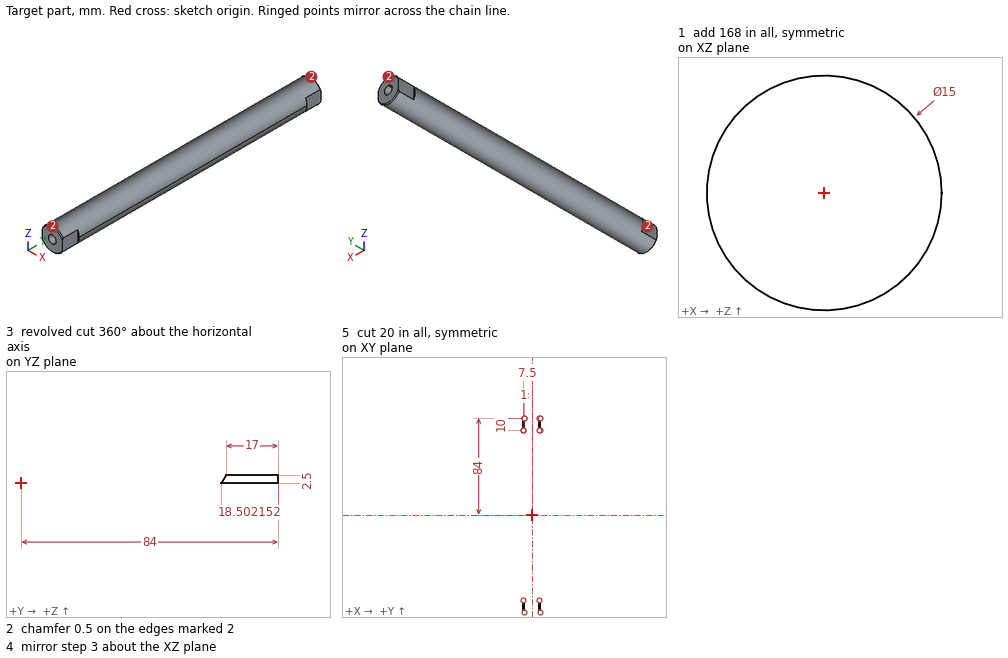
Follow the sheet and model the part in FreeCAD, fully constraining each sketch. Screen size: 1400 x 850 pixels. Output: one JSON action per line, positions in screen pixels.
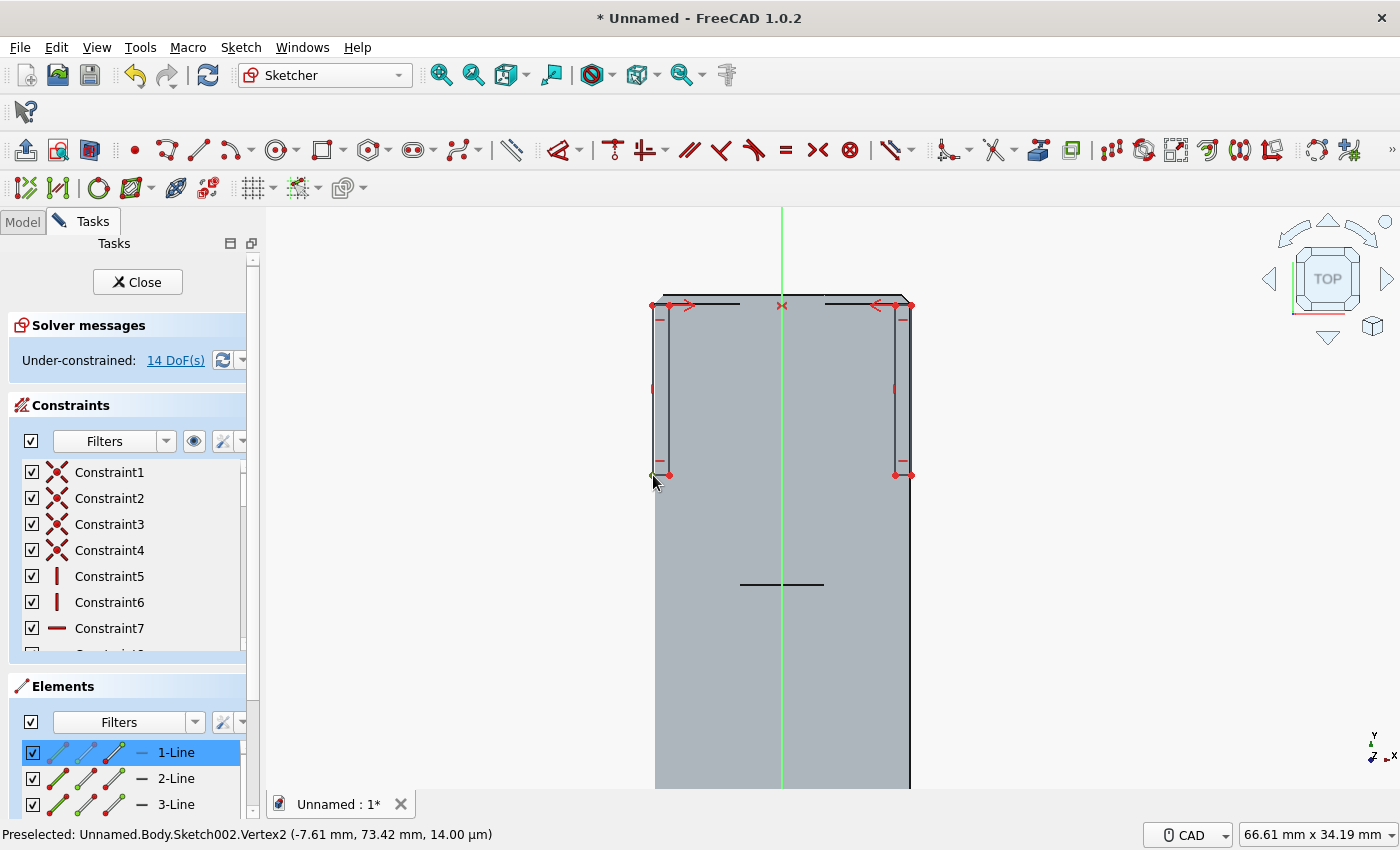
{"action": "left_click", "coordinate": [911, 475]}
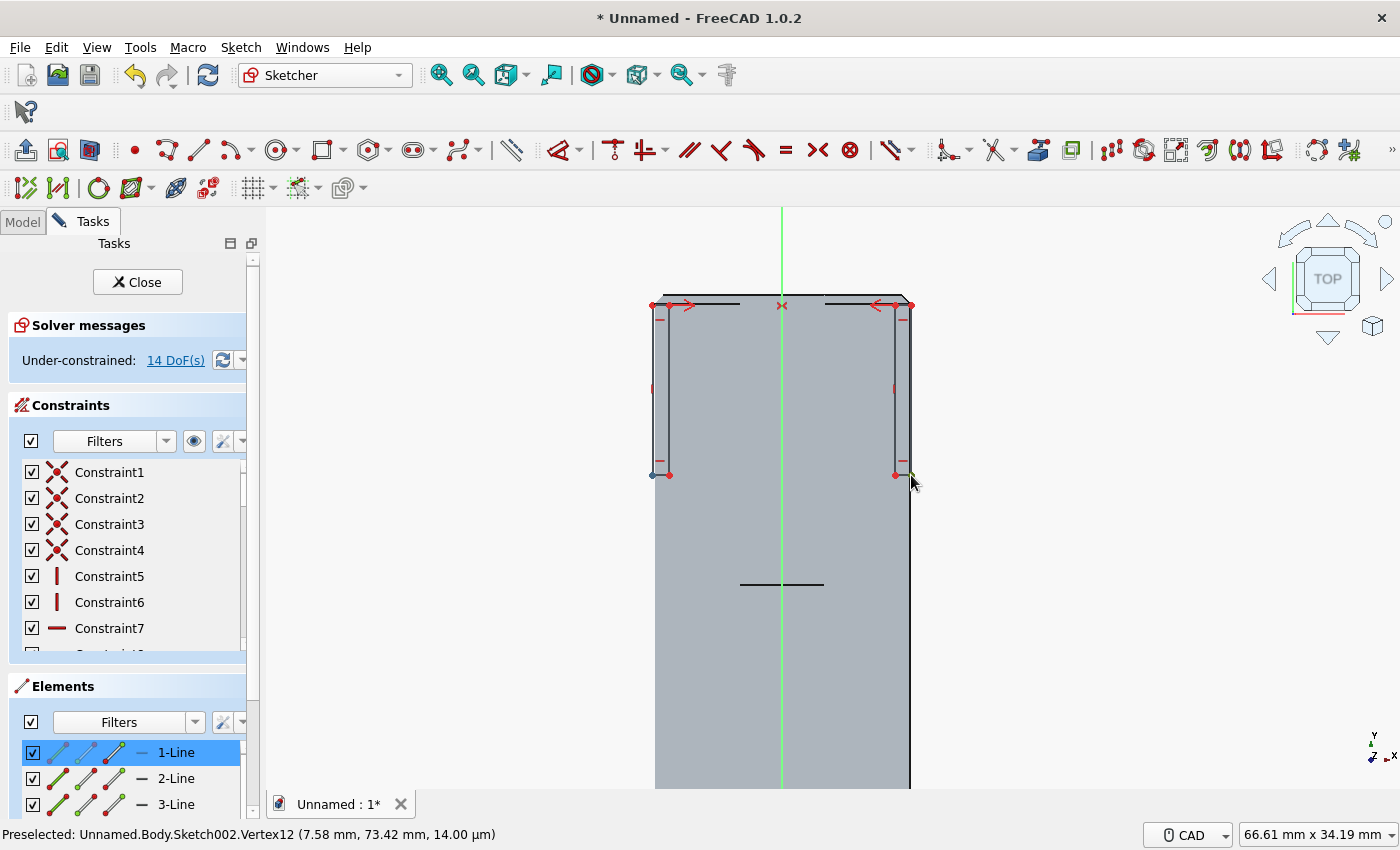
{"action": "left_click", "coordinate": [782, 723]}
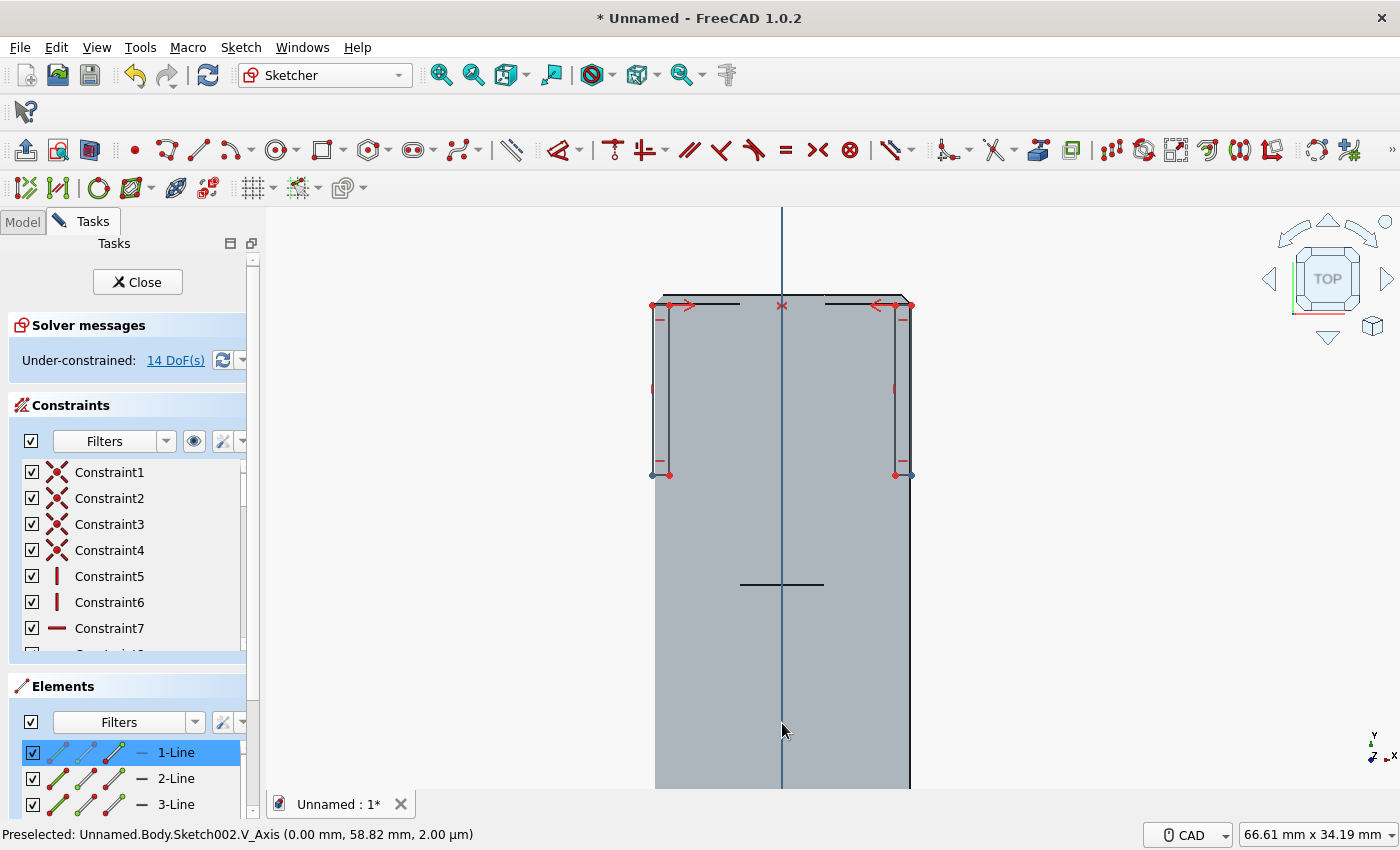
{"action": "left_click", "coordinate": [818, 150]}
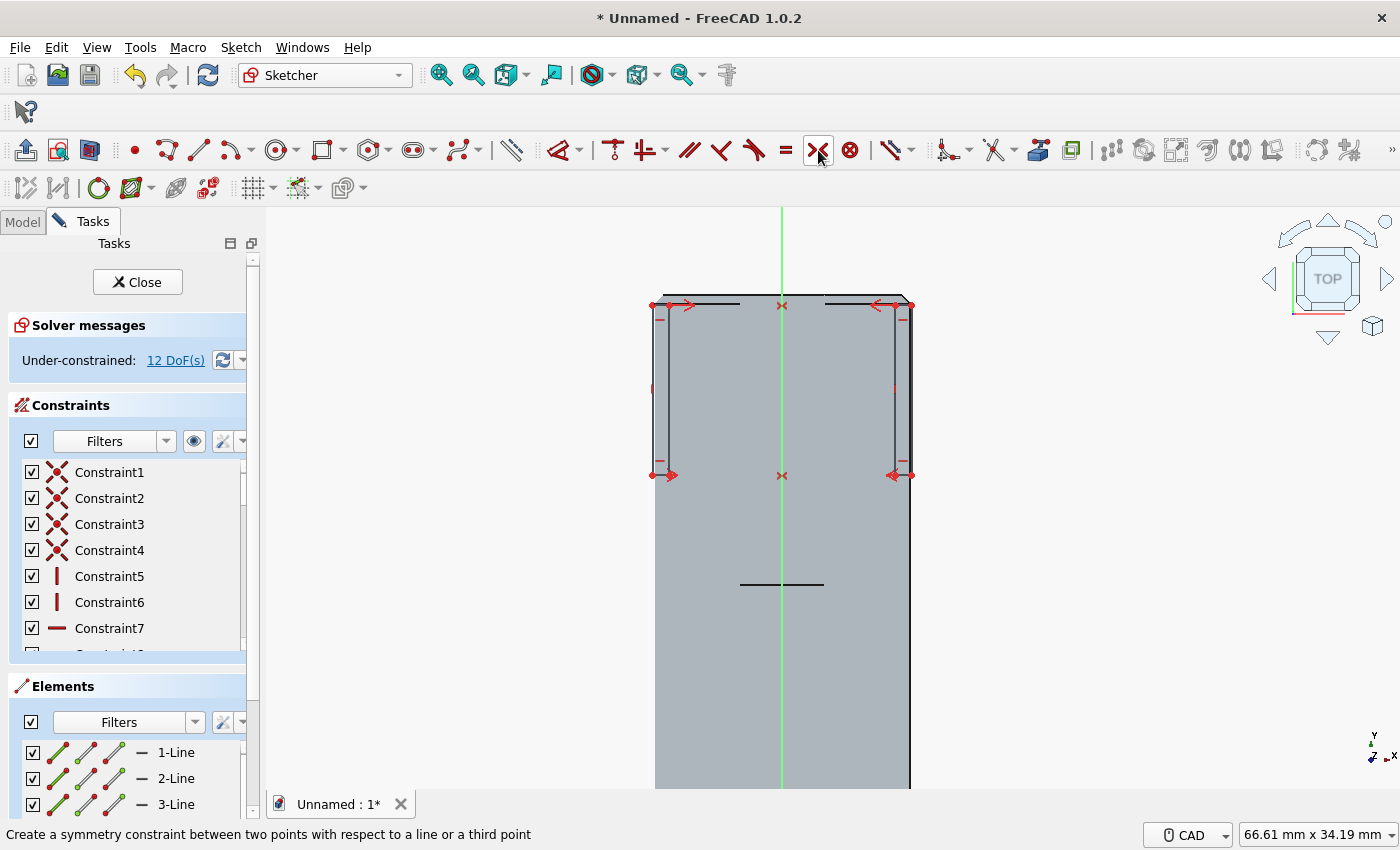
{"action": "left_click", "coordinate": [895, 475]}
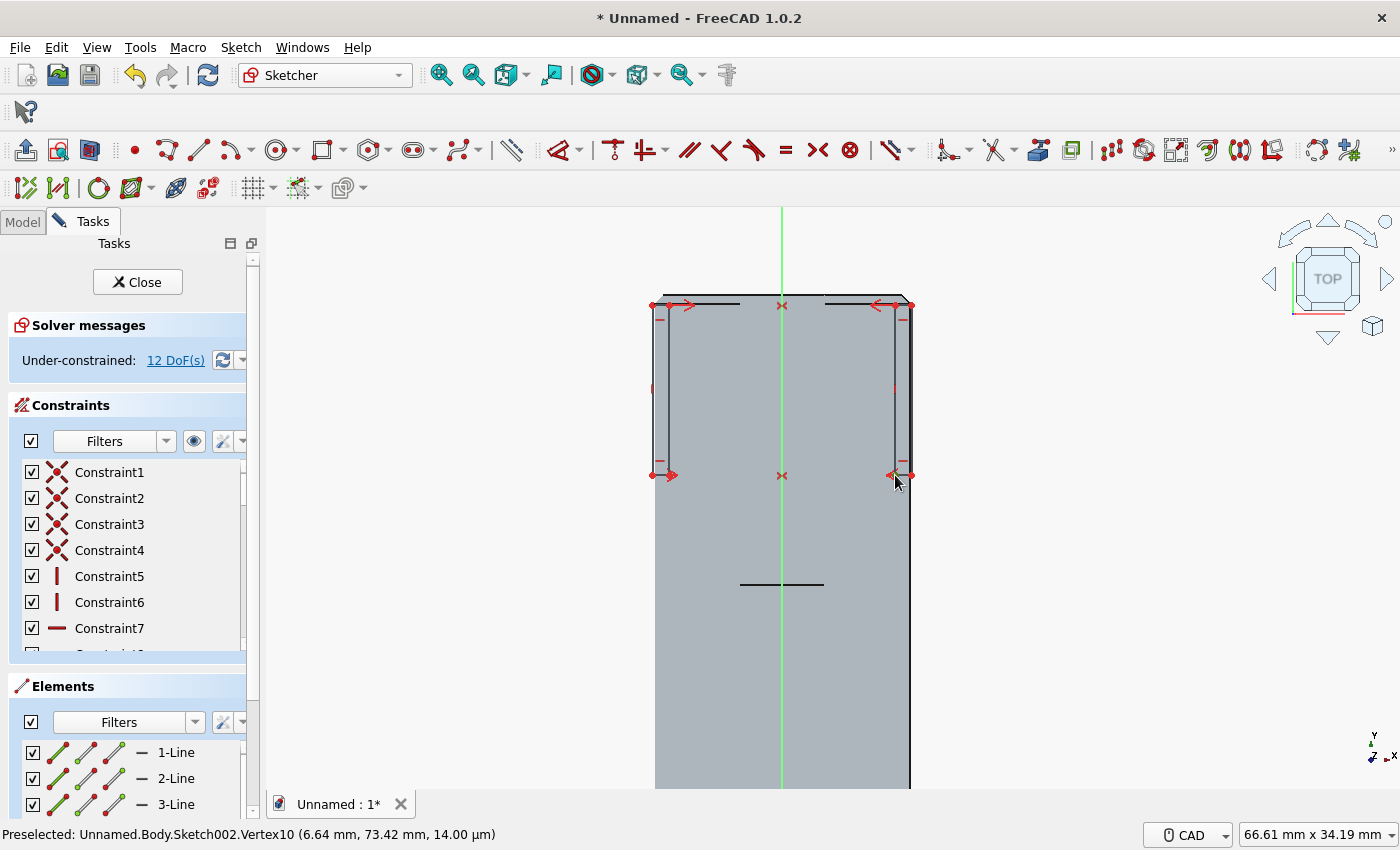
{"action": "scroll", "coordinate": [762, 306], "scroll_direction": "down", "scroll_amount": 10}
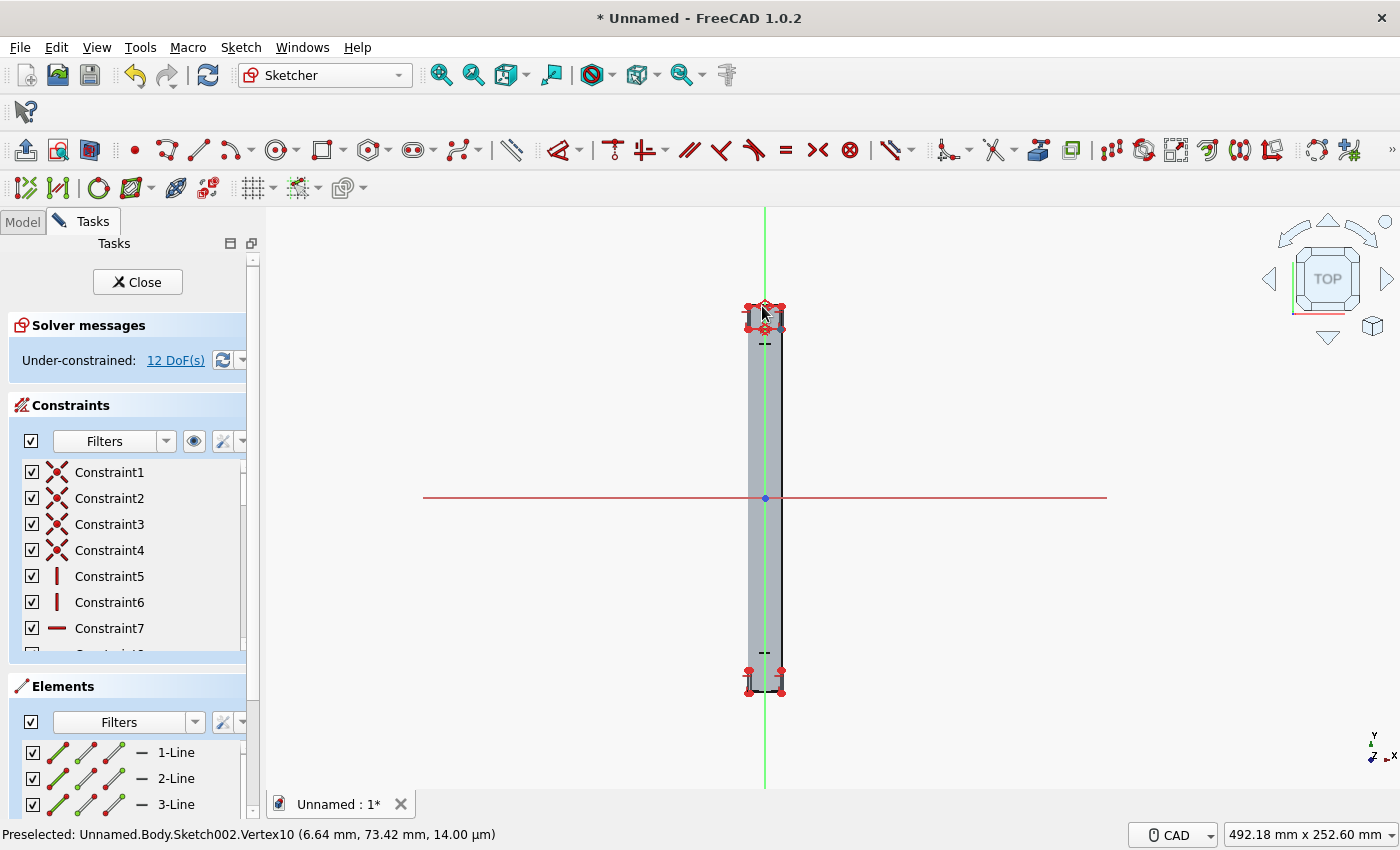
{"action": "scroll", "coordinate": [781, 670], "scroll_direction": "up", "scroll_amount": 10}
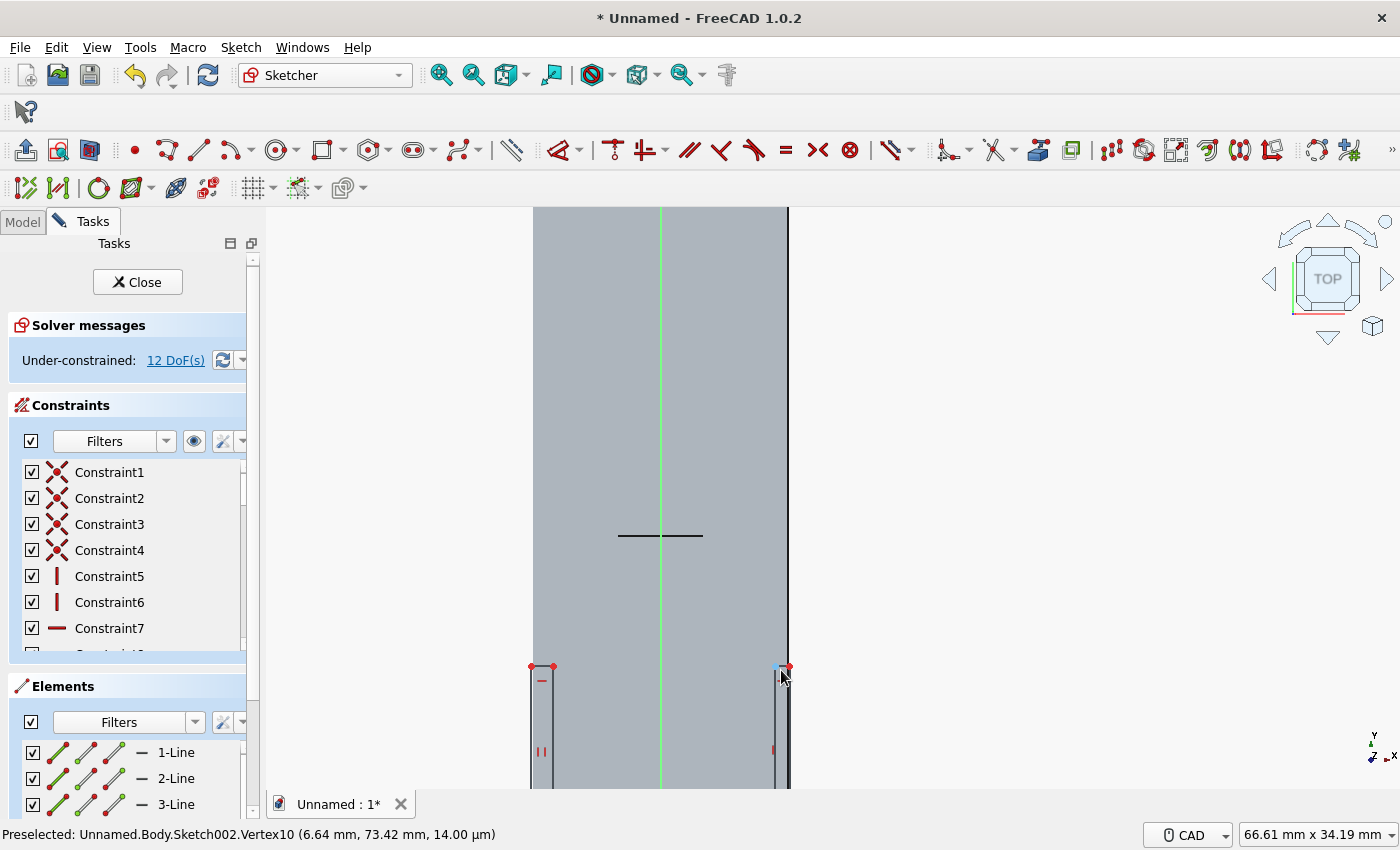
{"action": "left_click", "coordinate": [775, 666]}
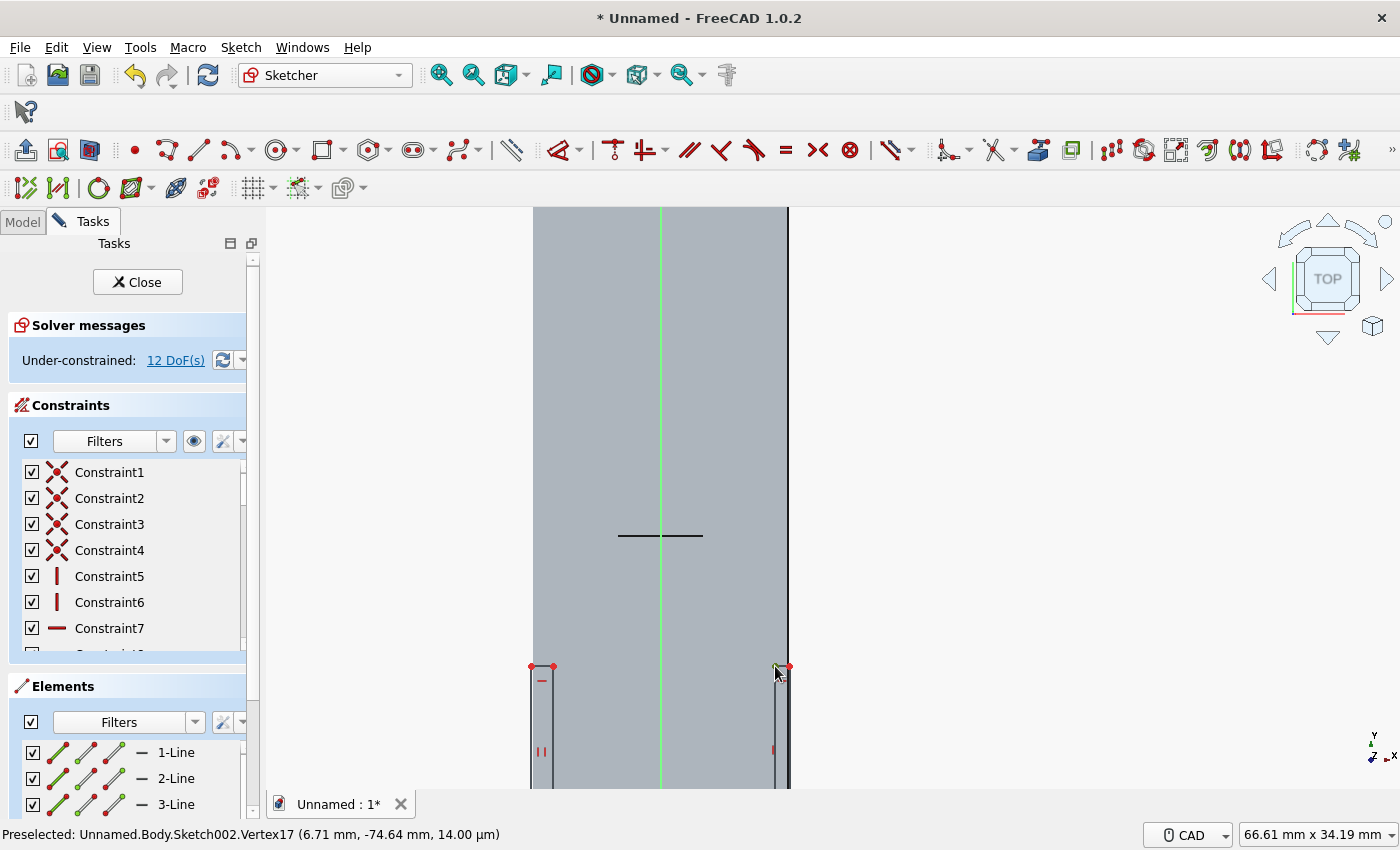
{"action": "scroll", "coordinate": [781, 671], "scroll_direction": "down", "scroll_amount": 10}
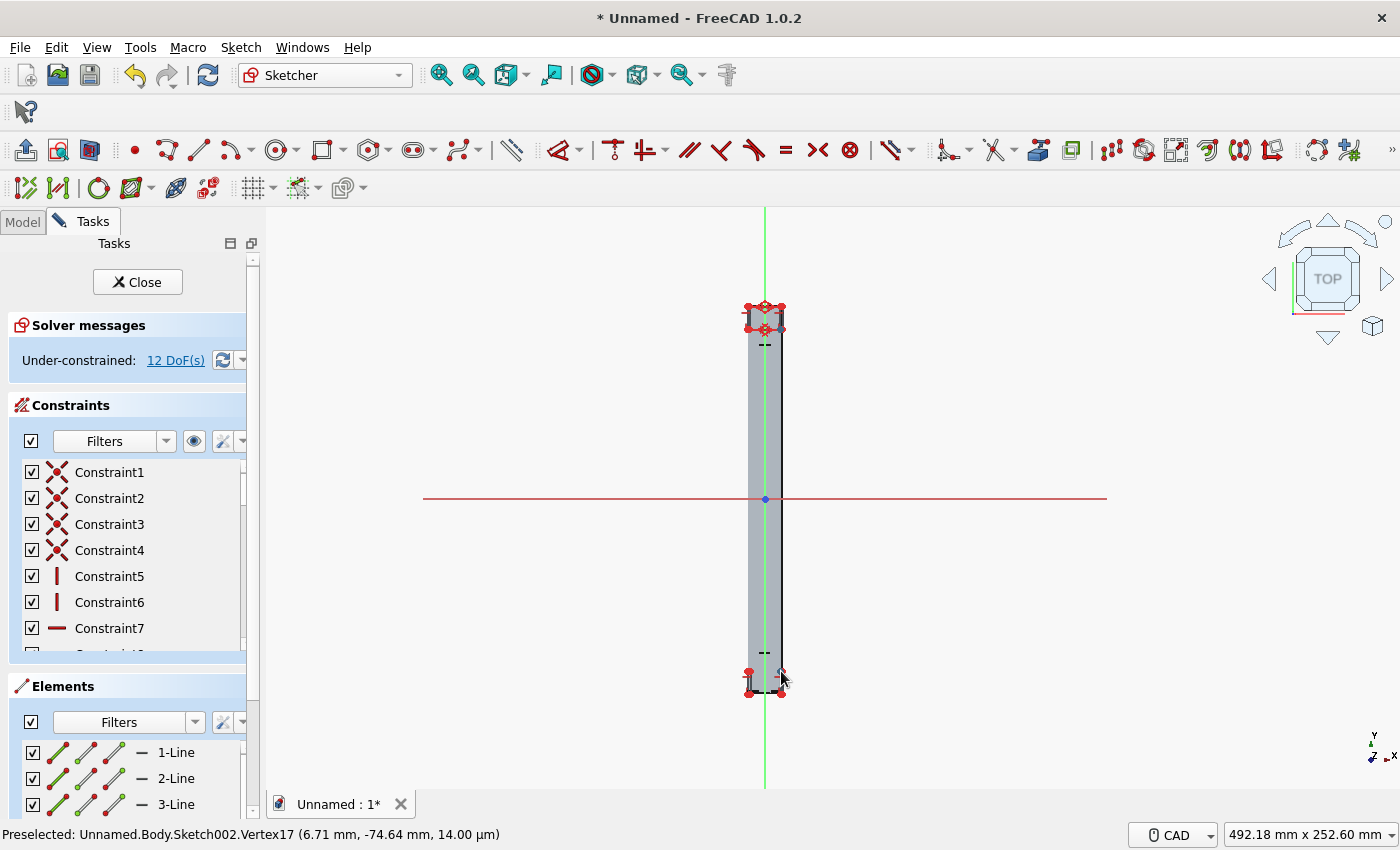
{"action": "left_click", "coordinate": [428, 499]}